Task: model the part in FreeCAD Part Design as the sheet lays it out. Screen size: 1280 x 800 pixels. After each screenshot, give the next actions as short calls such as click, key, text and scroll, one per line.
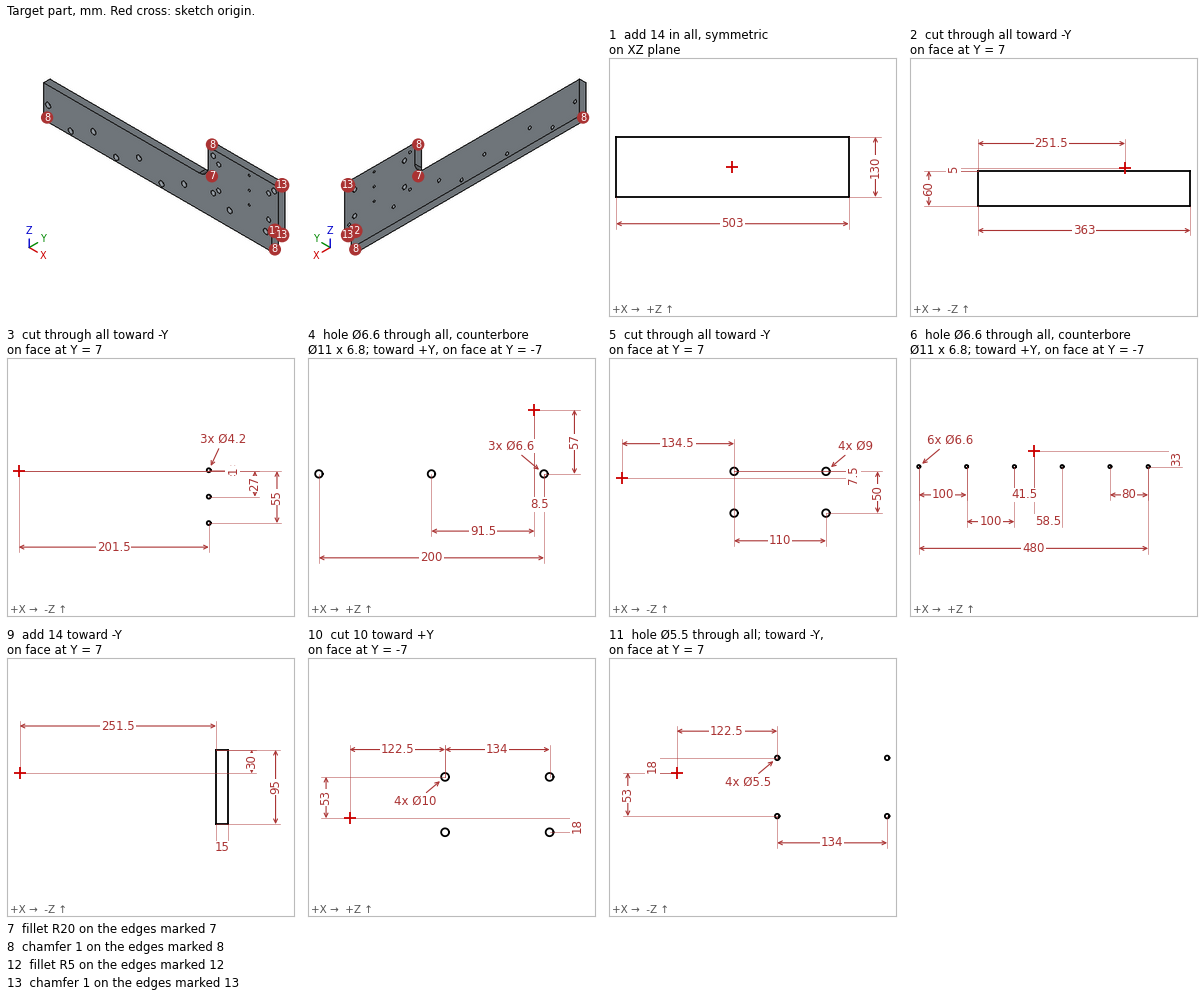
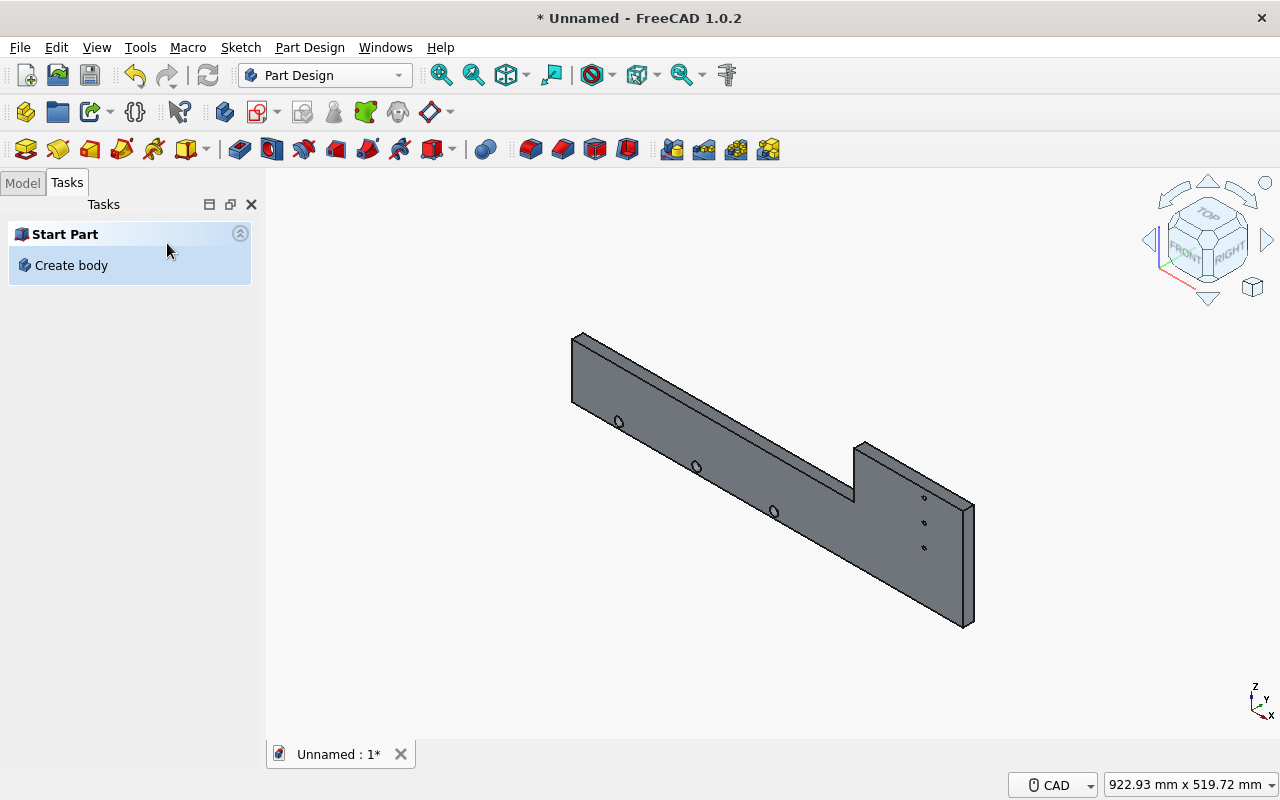
key(4)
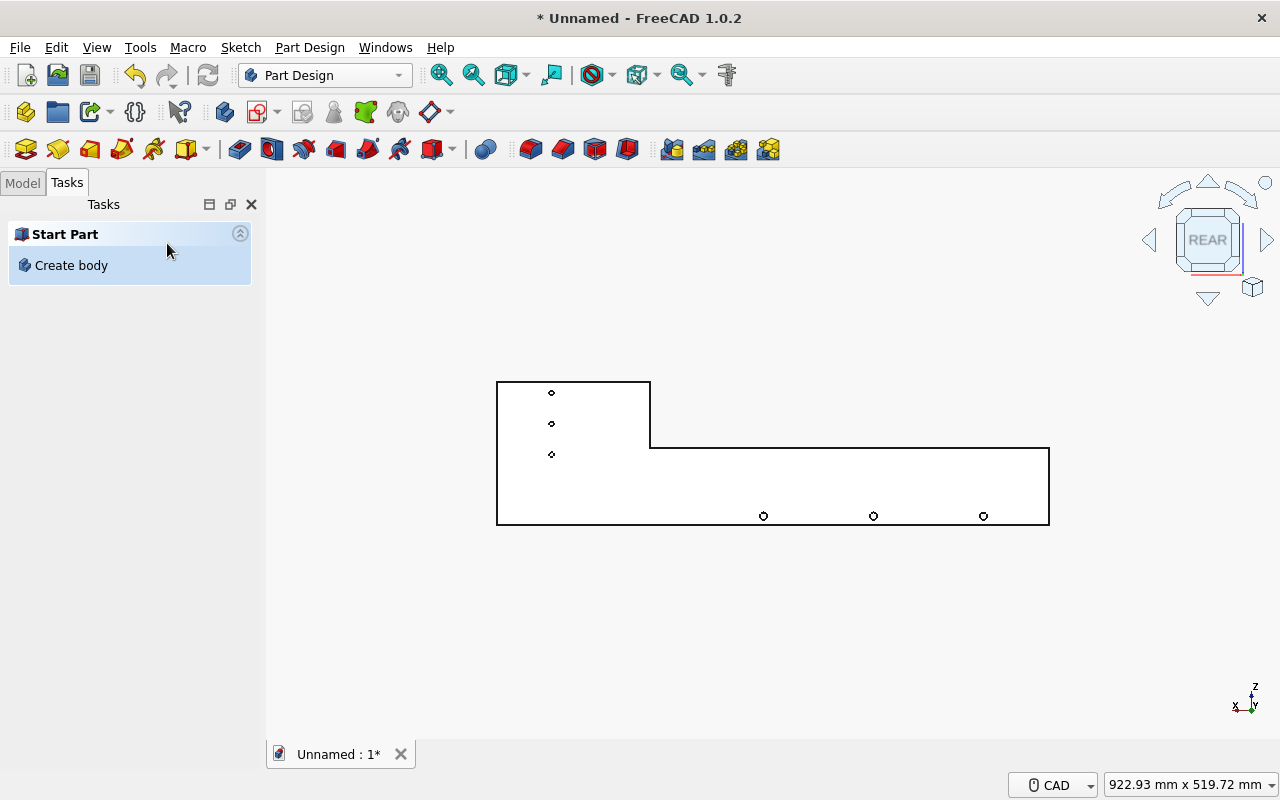
click(615, 473)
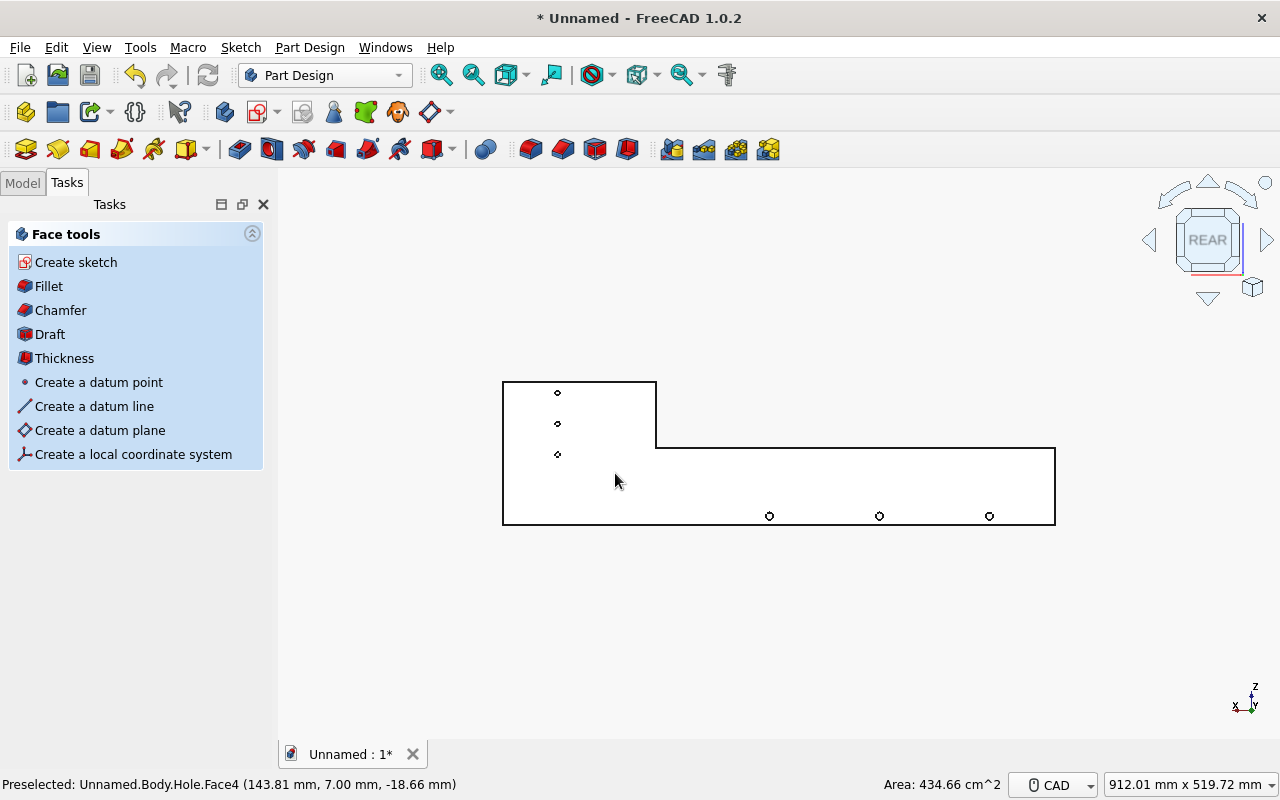
click(258, 112)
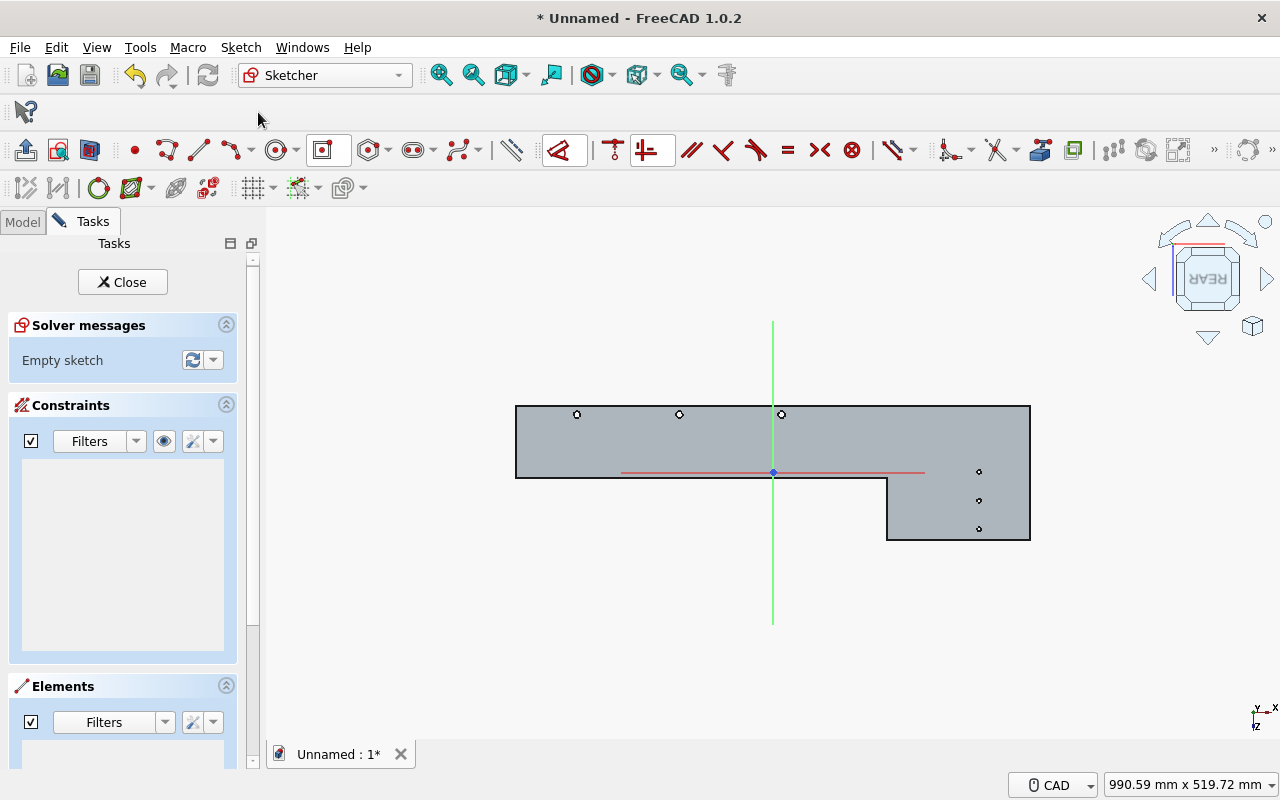
scroll(1060, 506, up, 4)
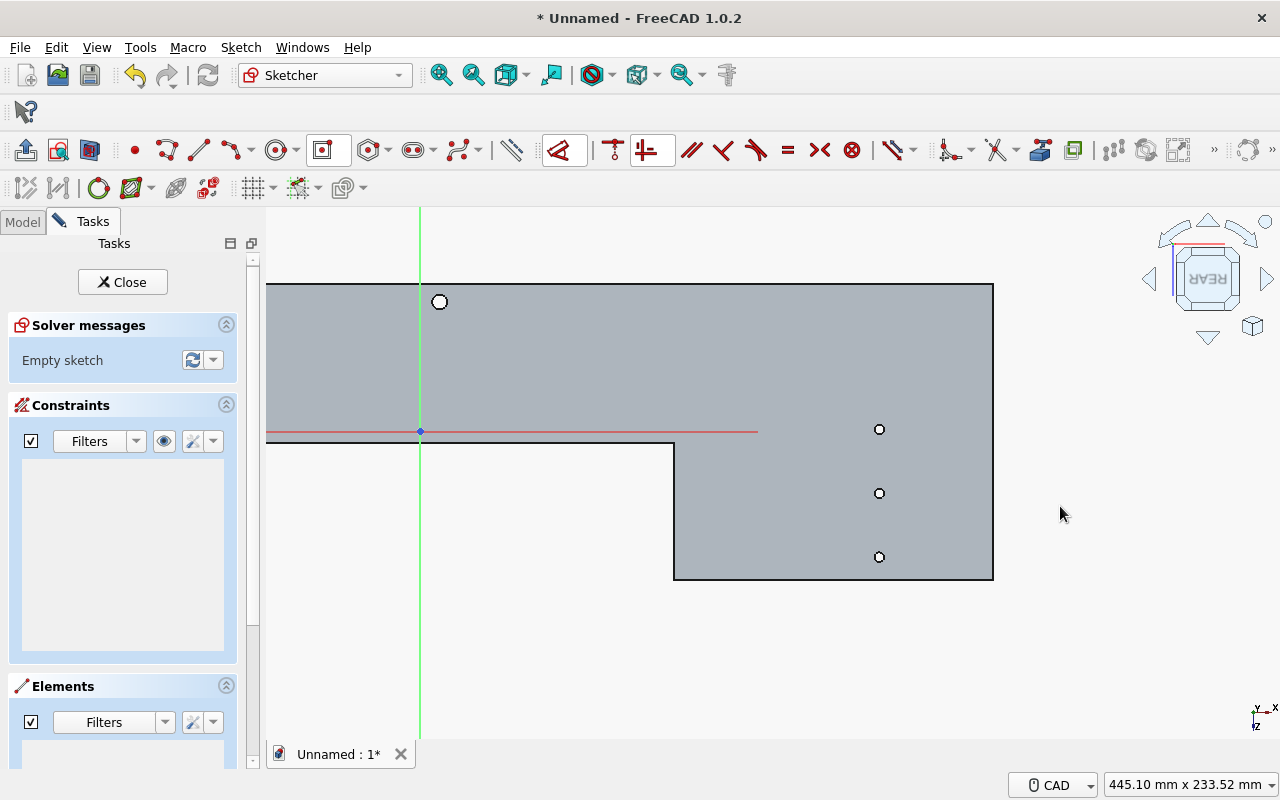
click(276, 150)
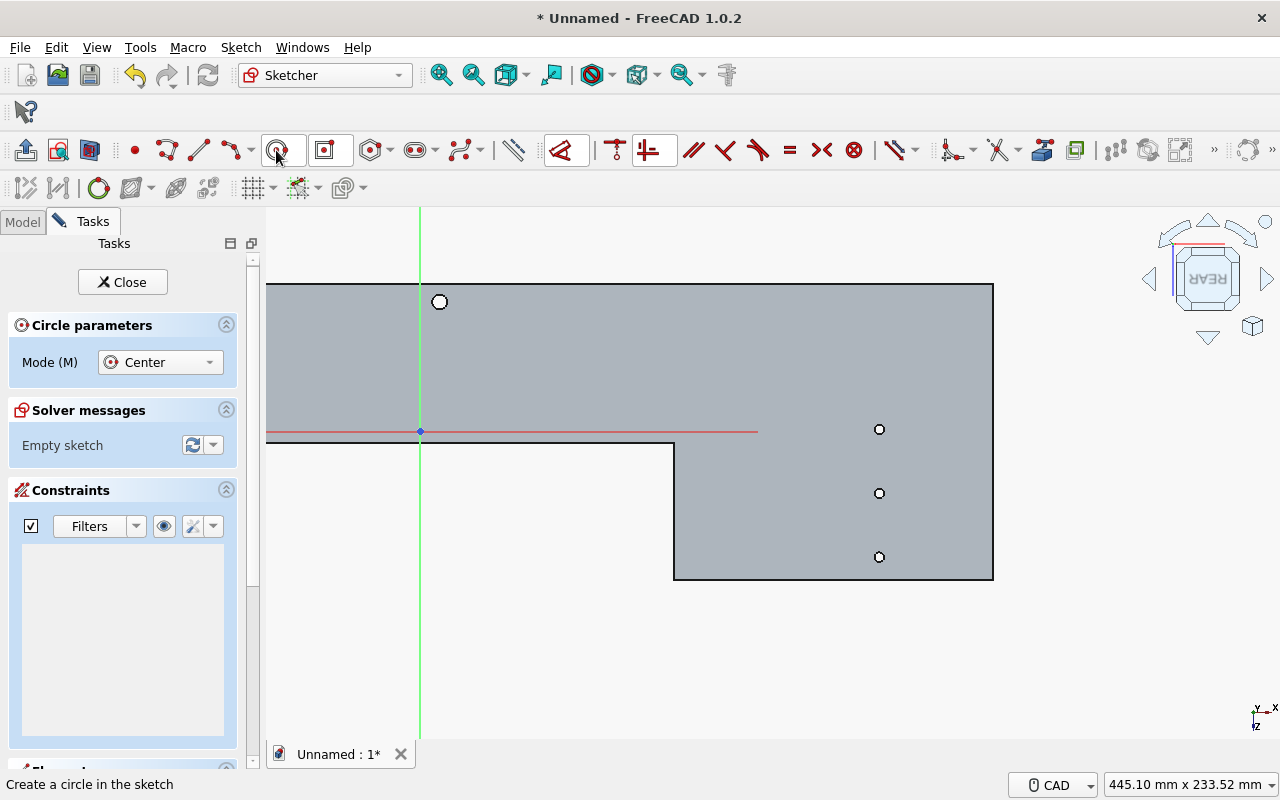
scroll(727, 415, up, 4)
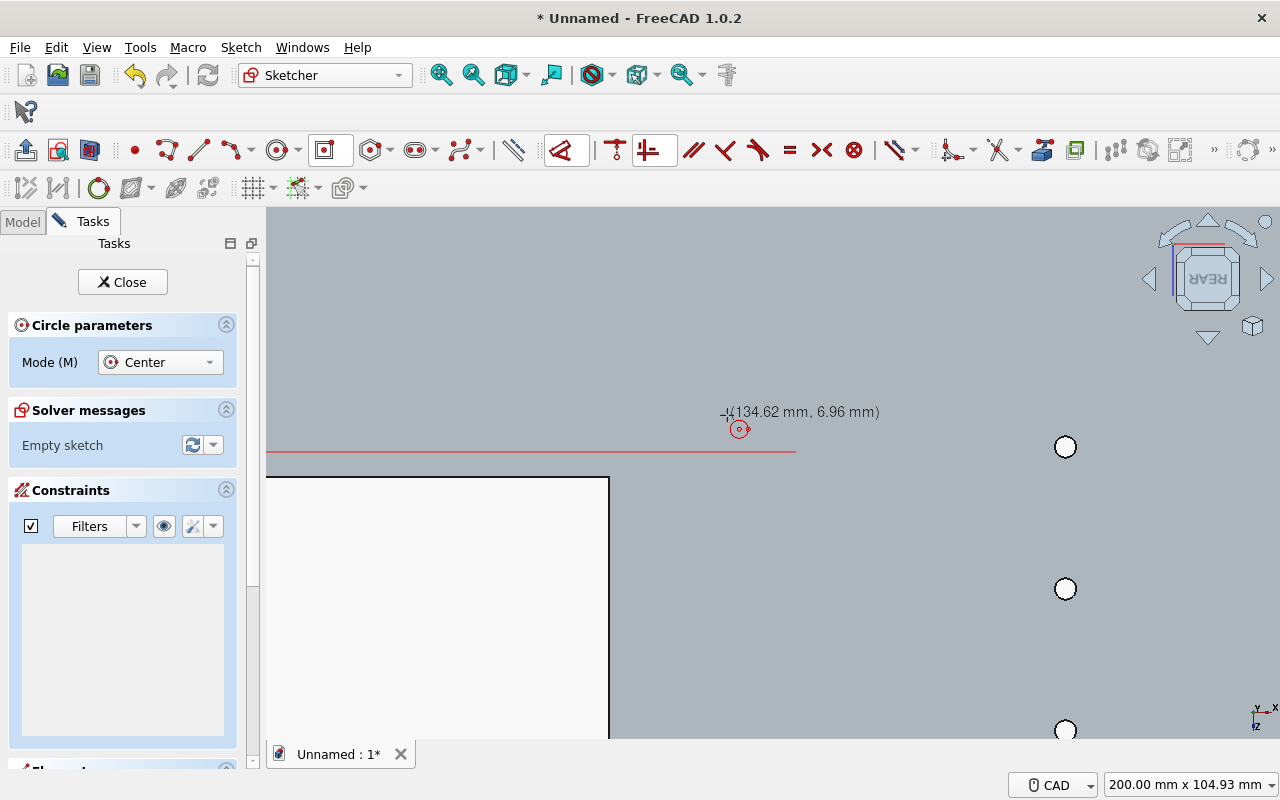
click(726, 414)
click(742, 398)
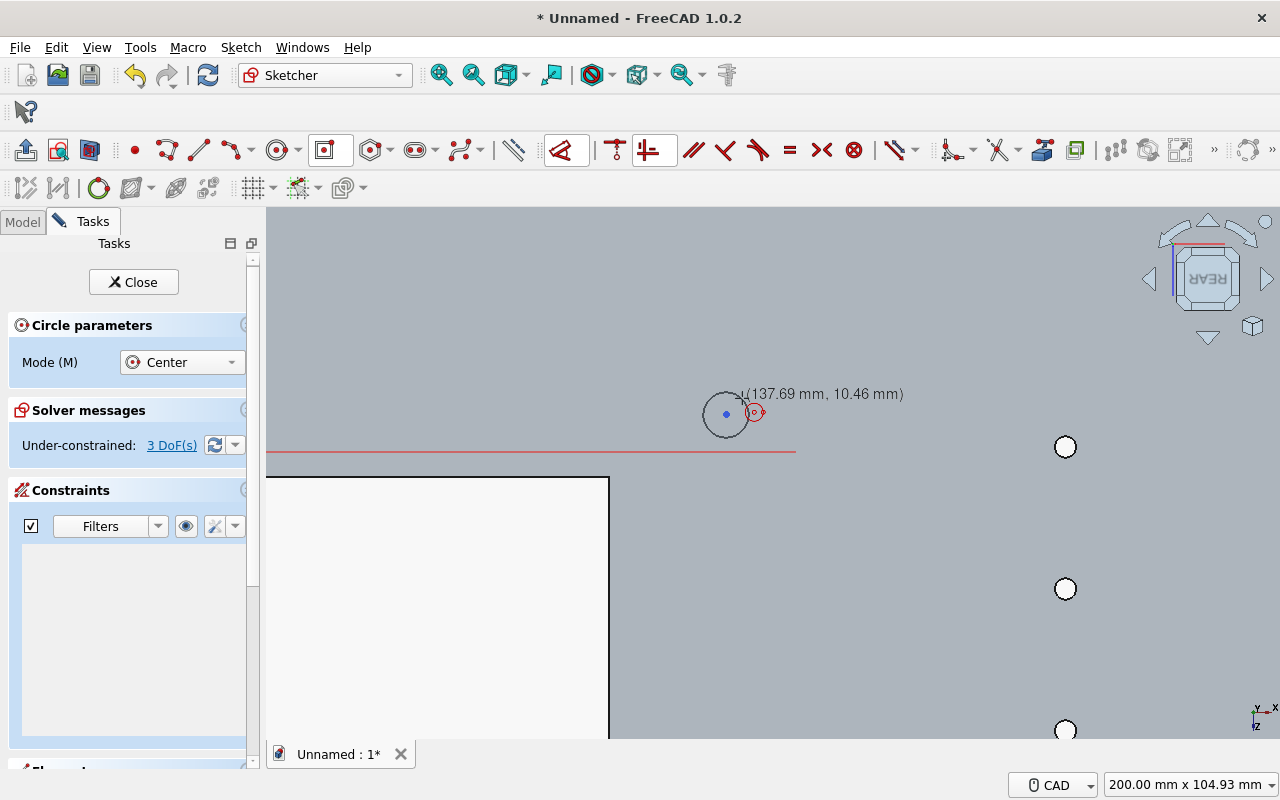
scroll(728, 418, down, 4)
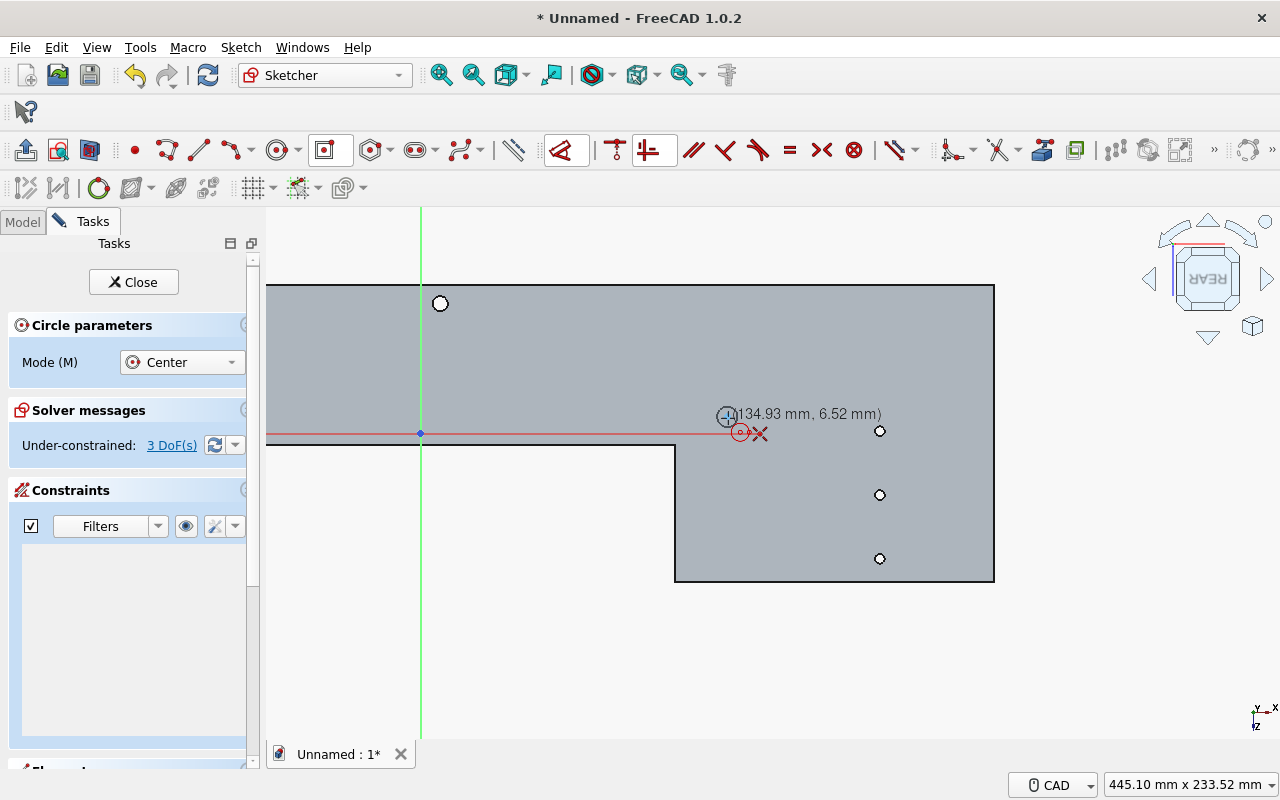
scroll(978, 530, up, 4)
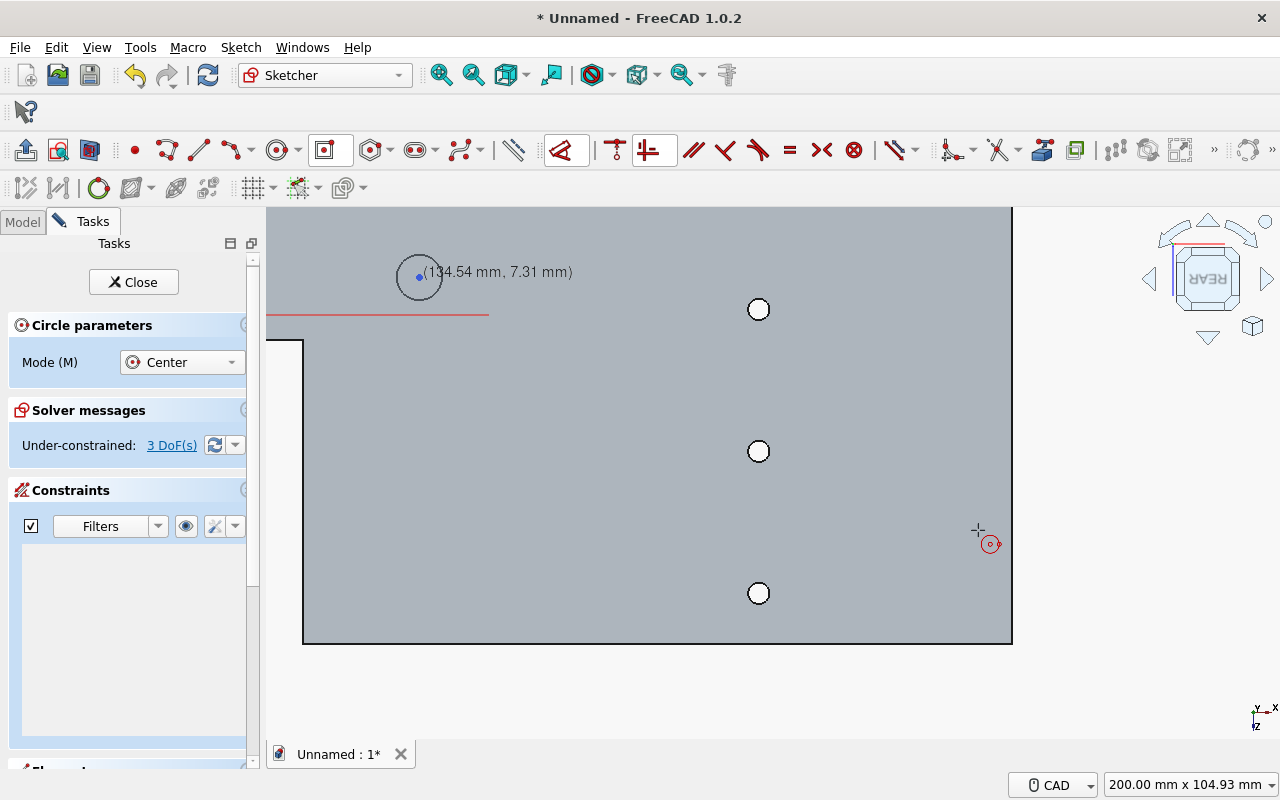
click(977, 530)
click(993, 514)